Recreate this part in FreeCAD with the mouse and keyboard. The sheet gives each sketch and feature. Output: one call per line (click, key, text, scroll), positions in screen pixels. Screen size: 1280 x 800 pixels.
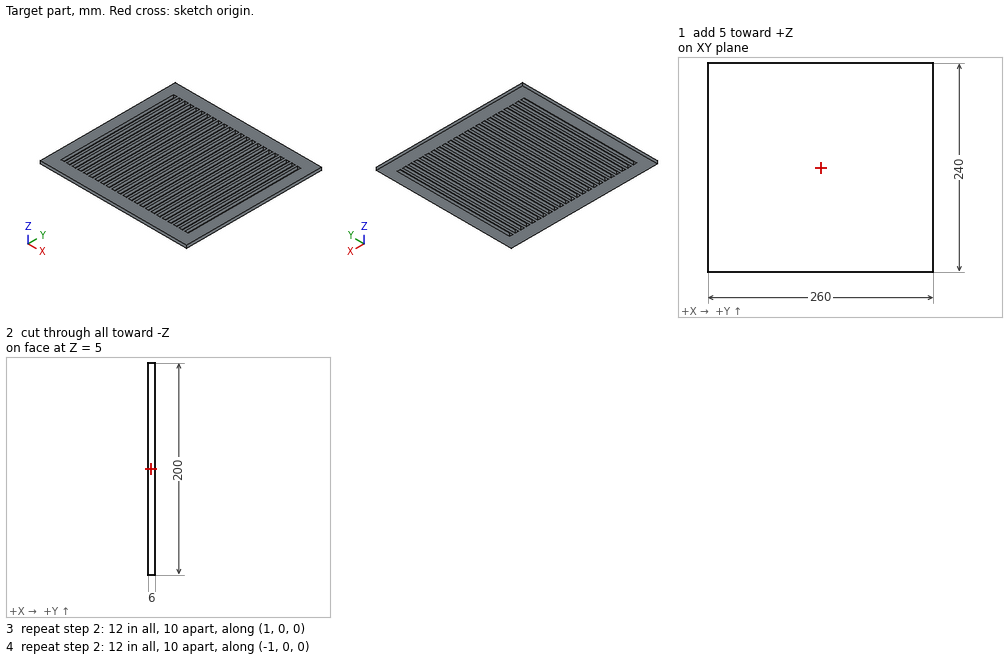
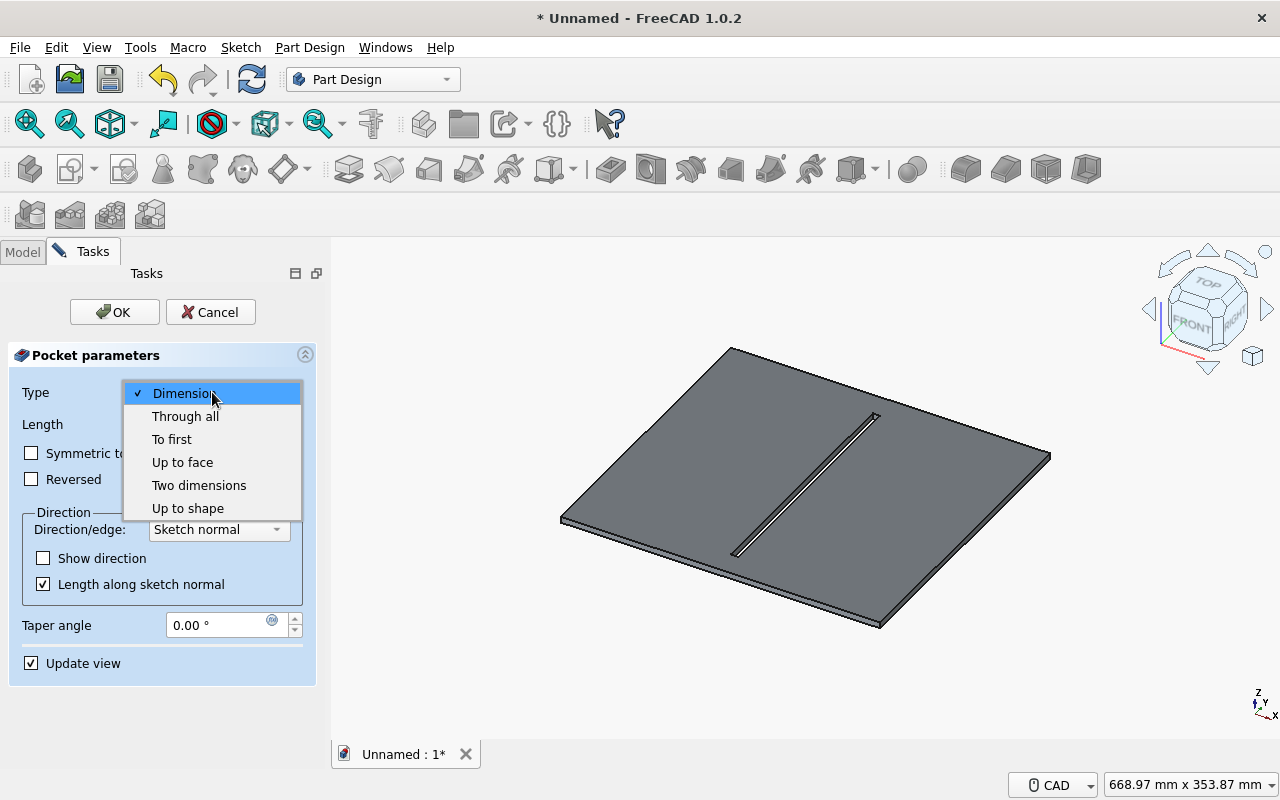
click(212, 416)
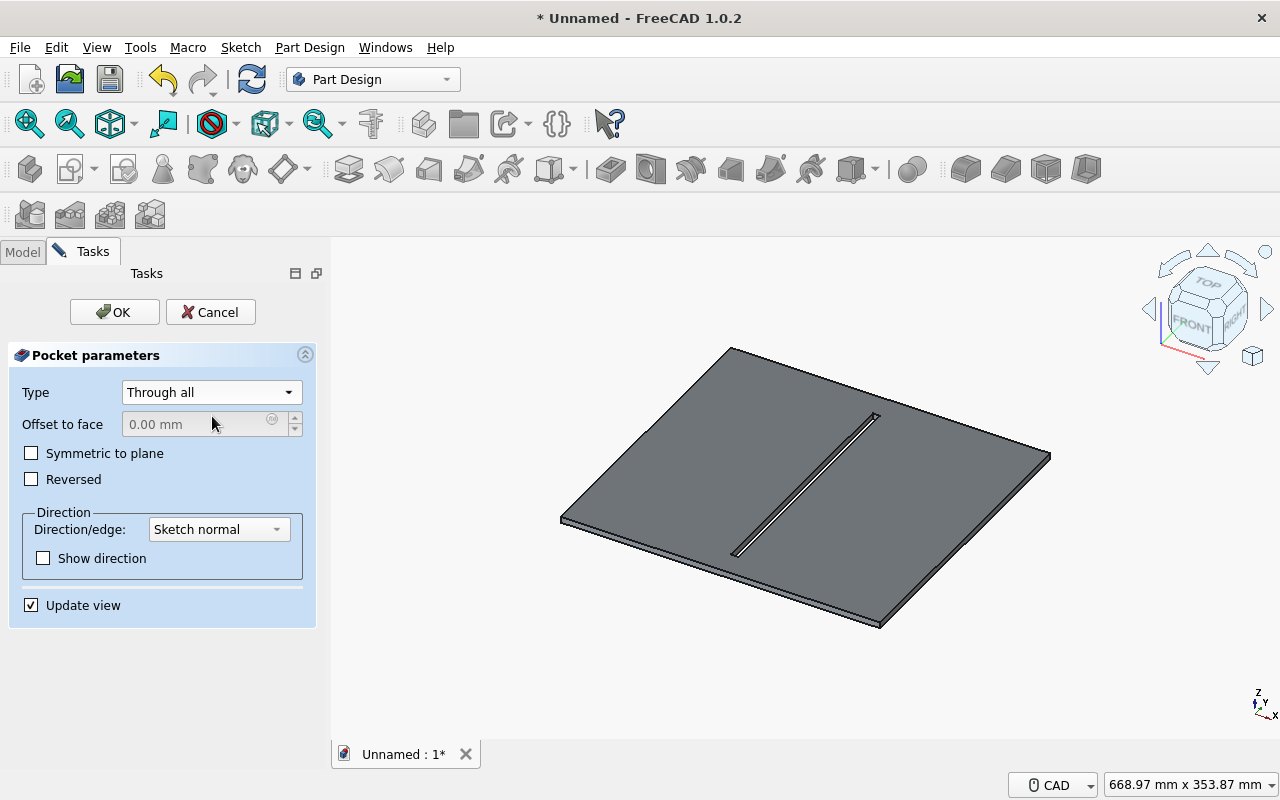
click(115, 312)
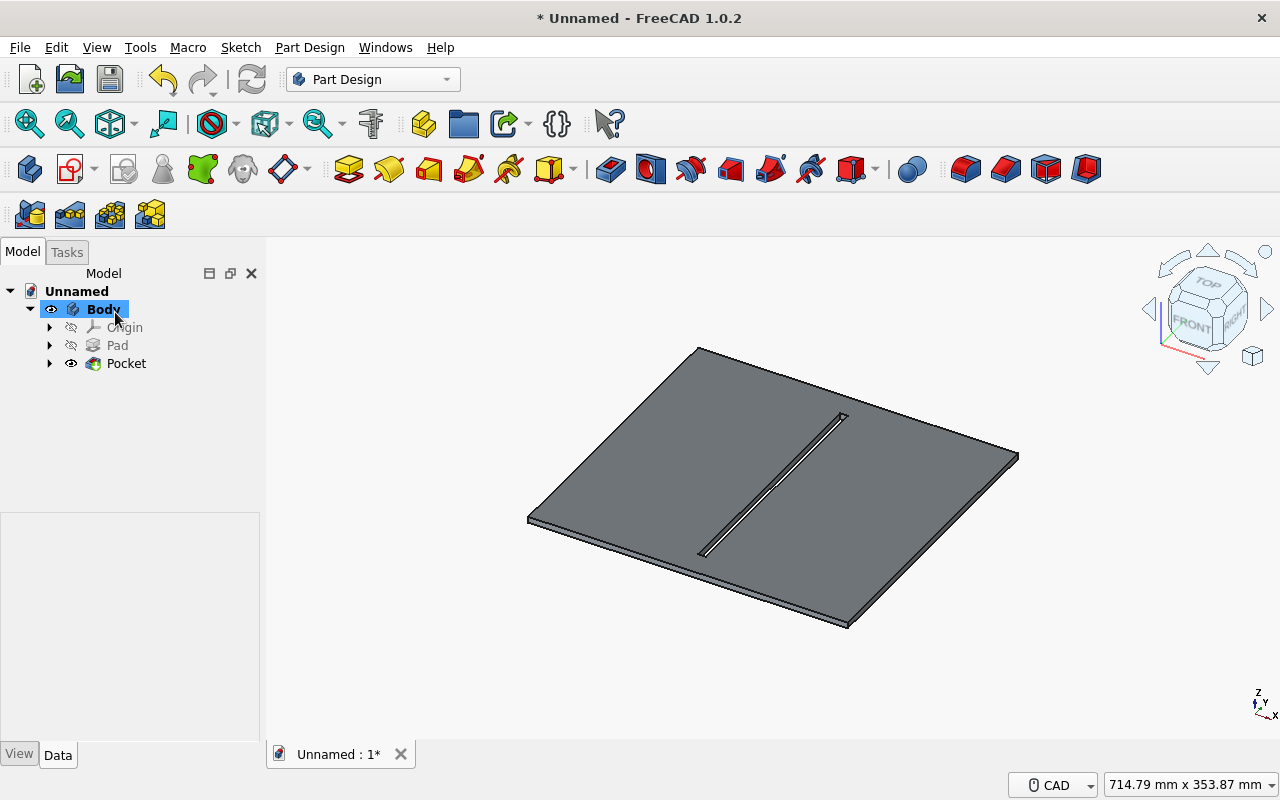
click(116, 363)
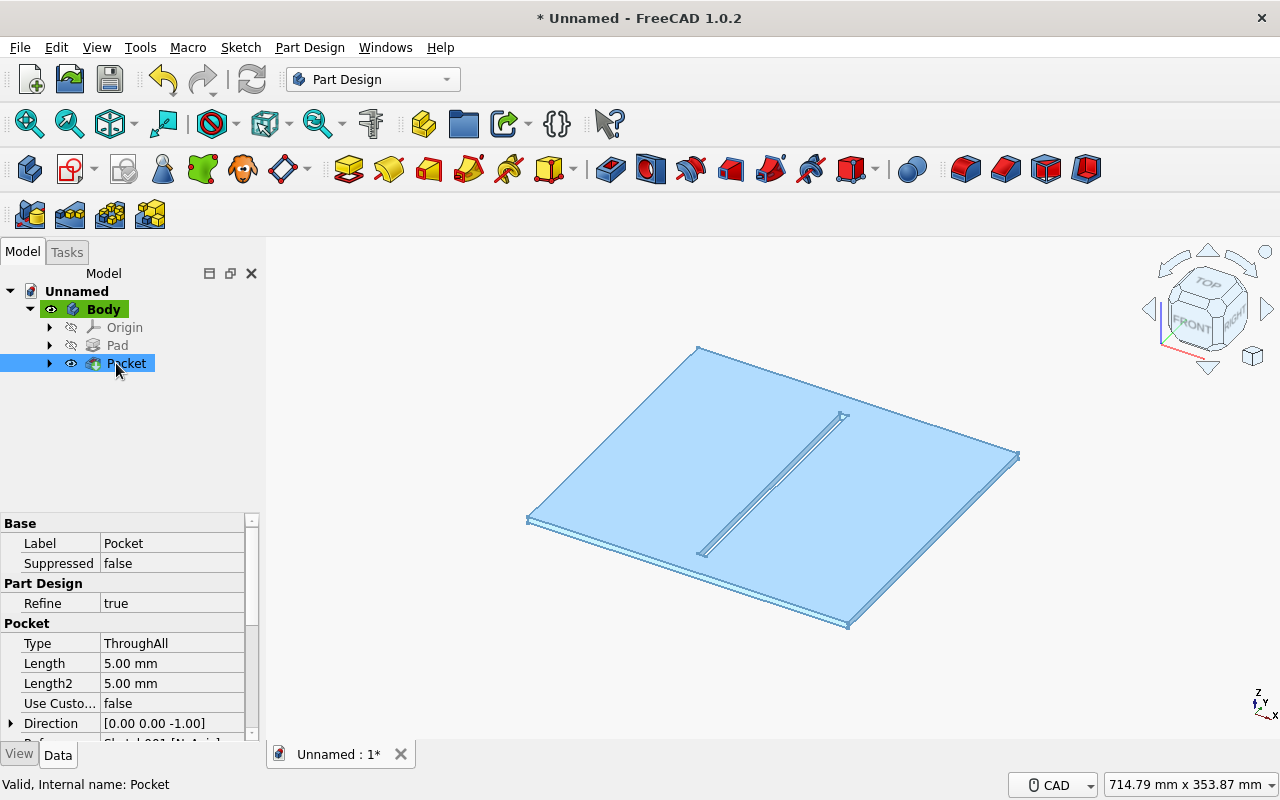
click(70, 214)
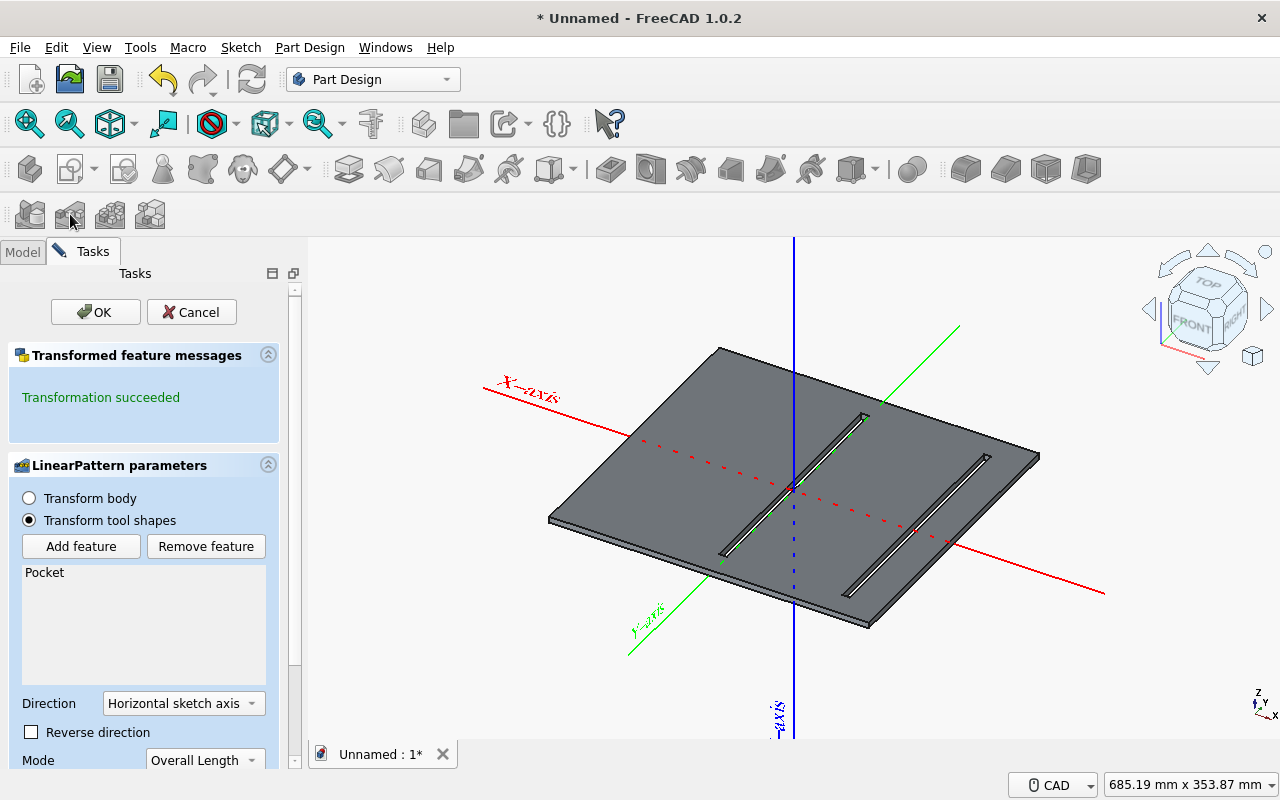
click(184, 704)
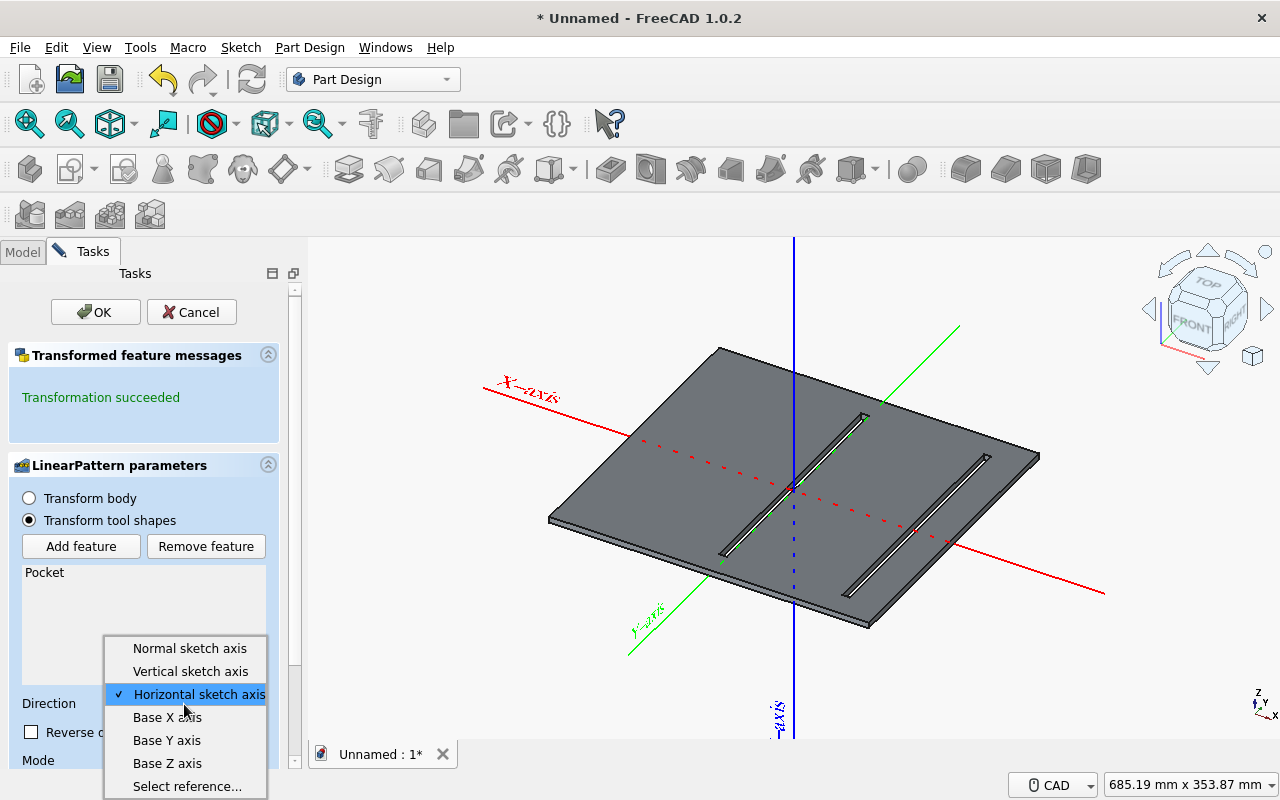
click(184, 718)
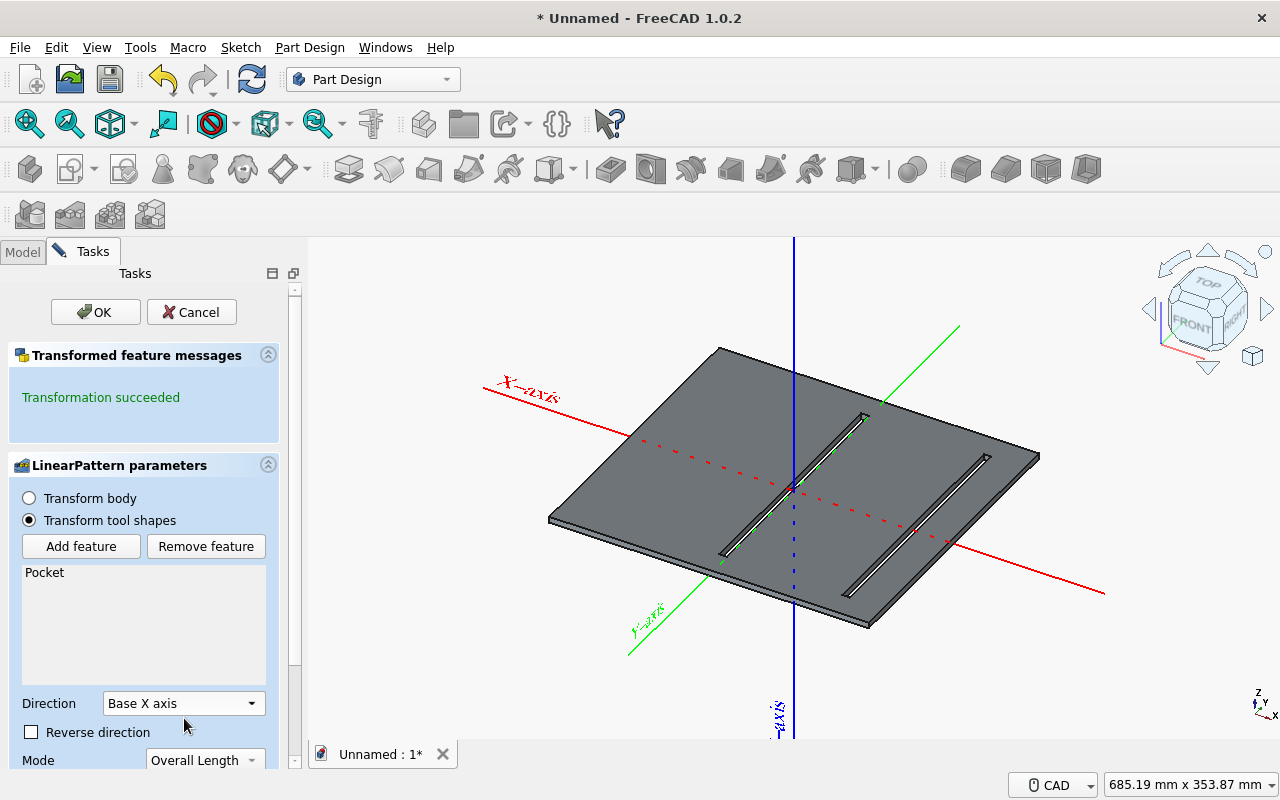
scroll(295, 526, down, 2)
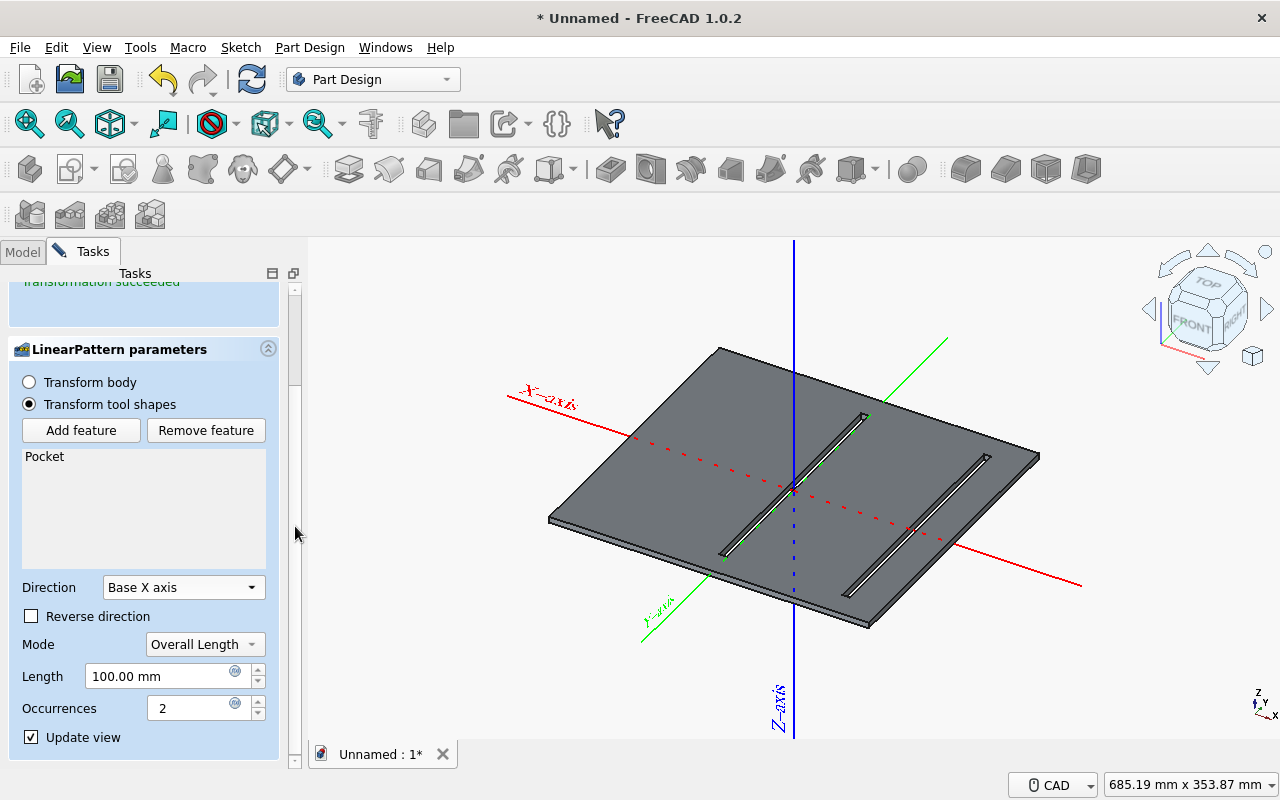
click(206, 644)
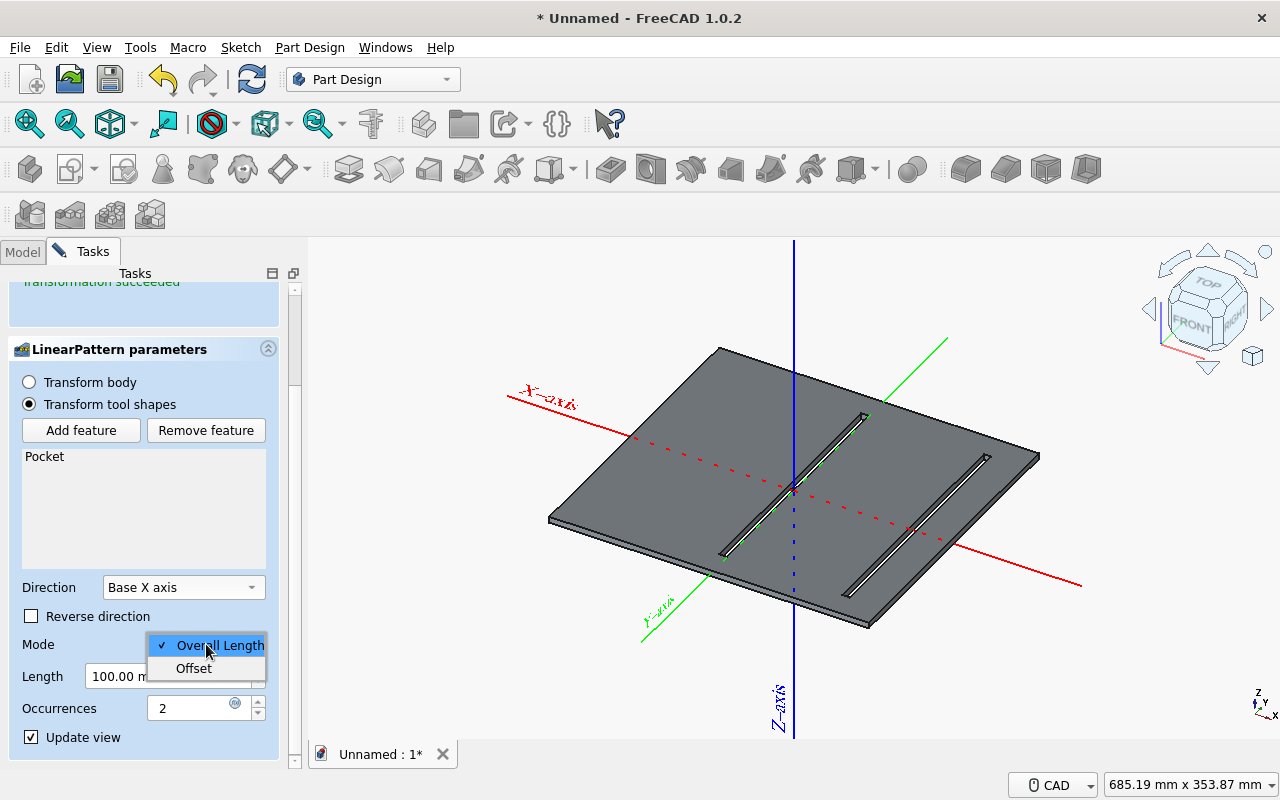
click(206, 668)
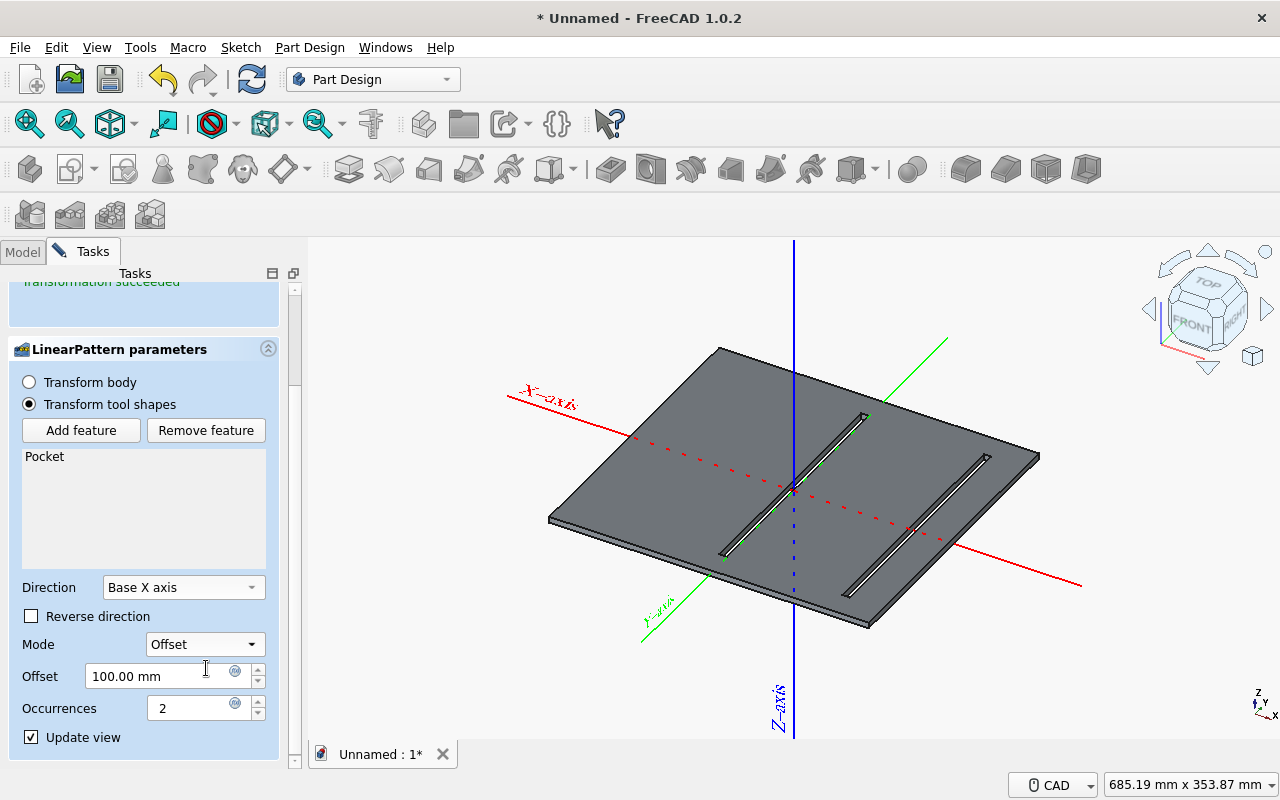
triple_click(168, 676)